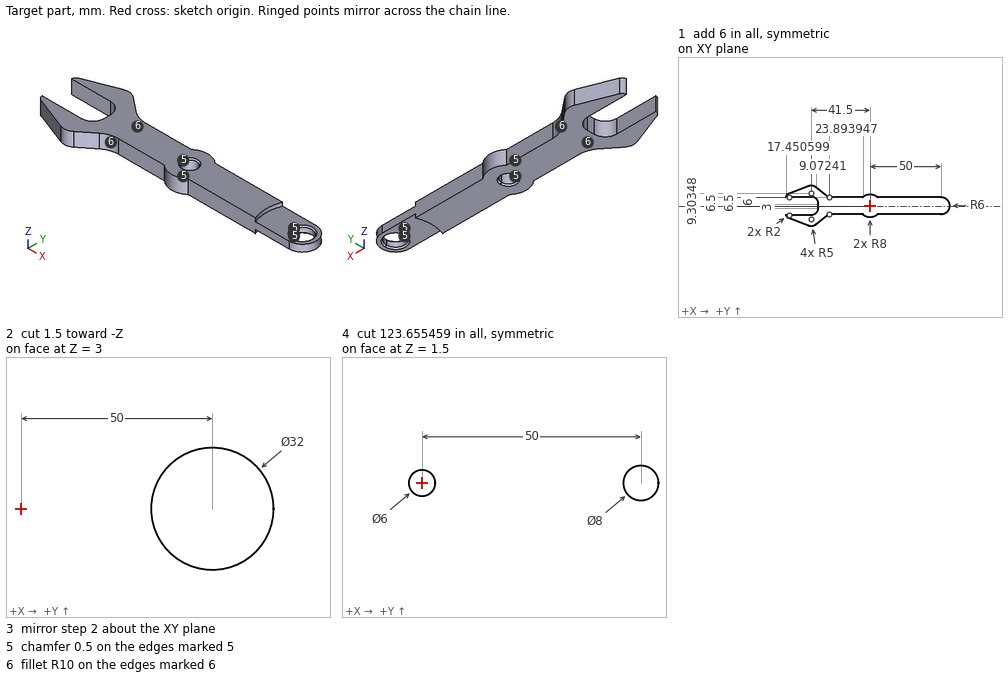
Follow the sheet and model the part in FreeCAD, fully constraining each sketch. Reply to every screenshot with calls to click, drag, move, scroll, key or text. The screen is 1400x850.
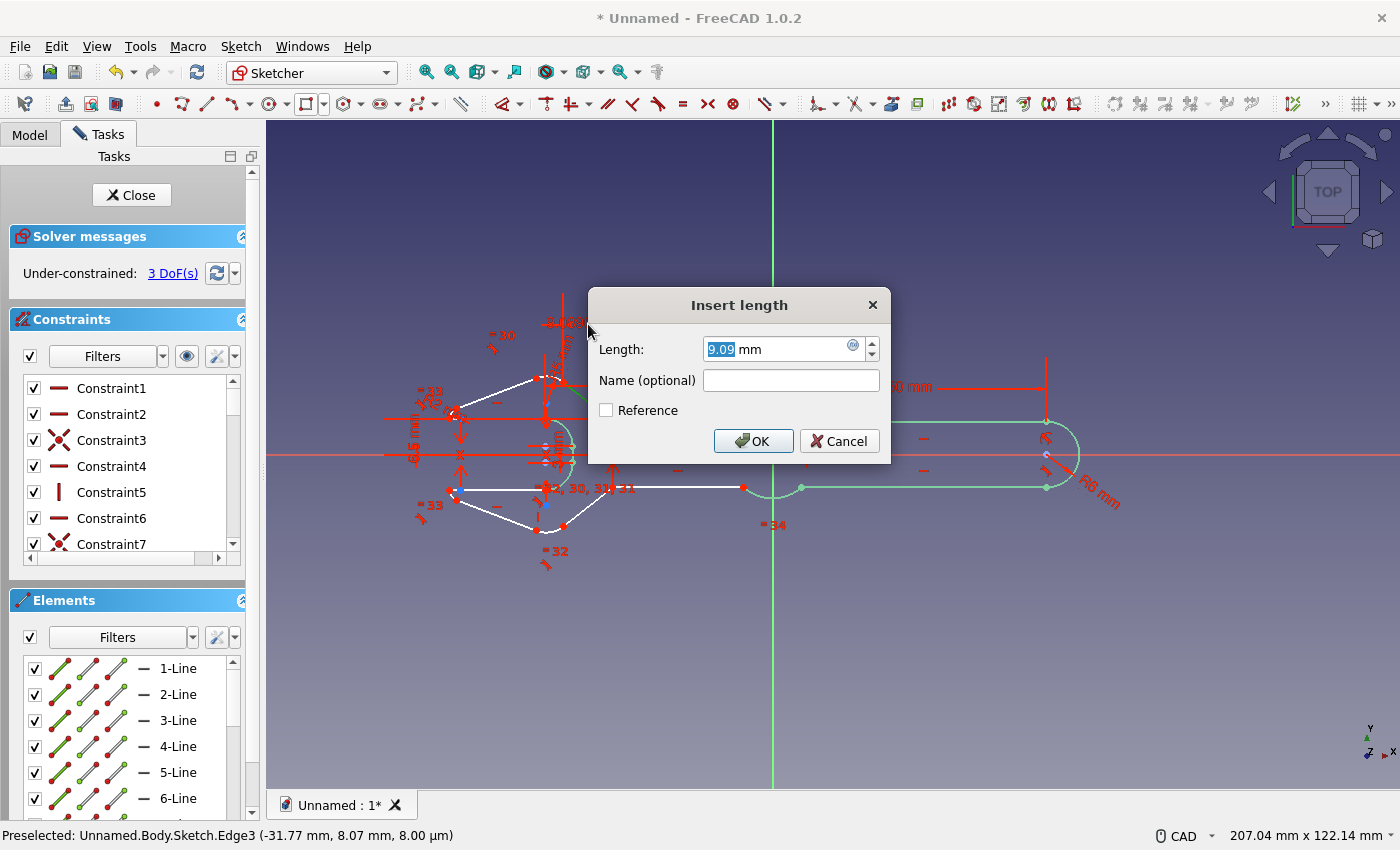
text(9.07241)
key(Return)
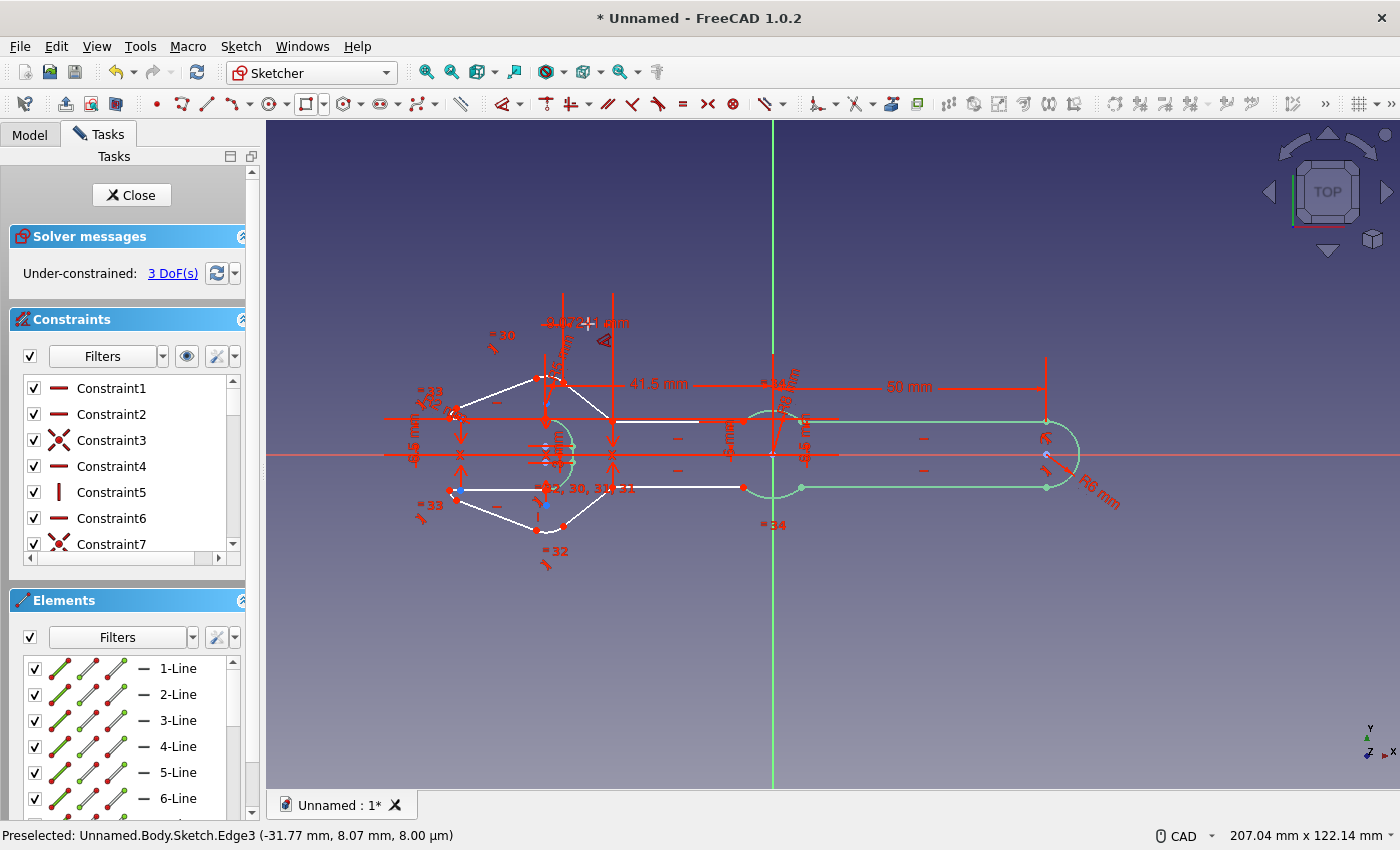
click(546, 404)
click(488, 441)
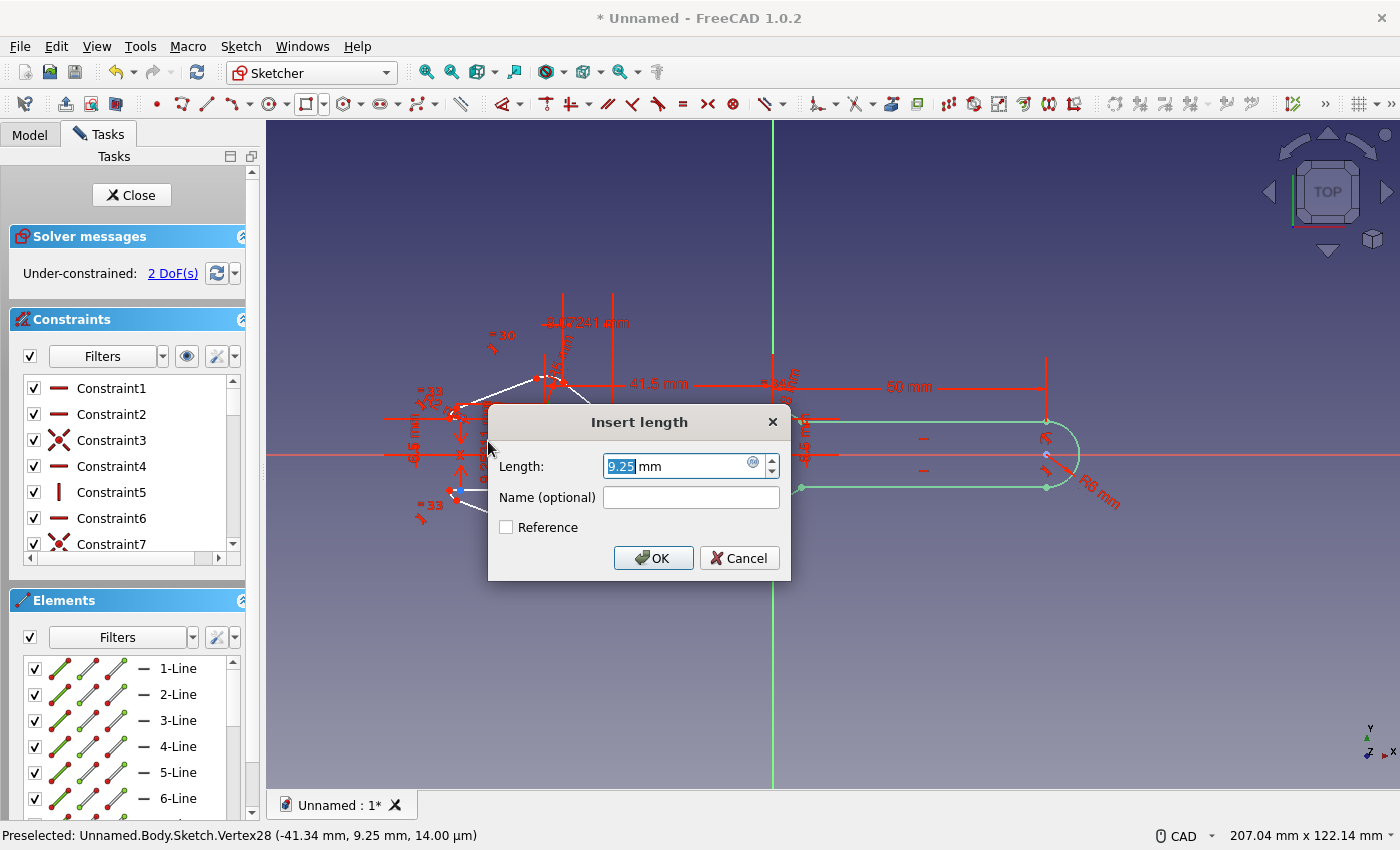
text(9.30348)
key(Return)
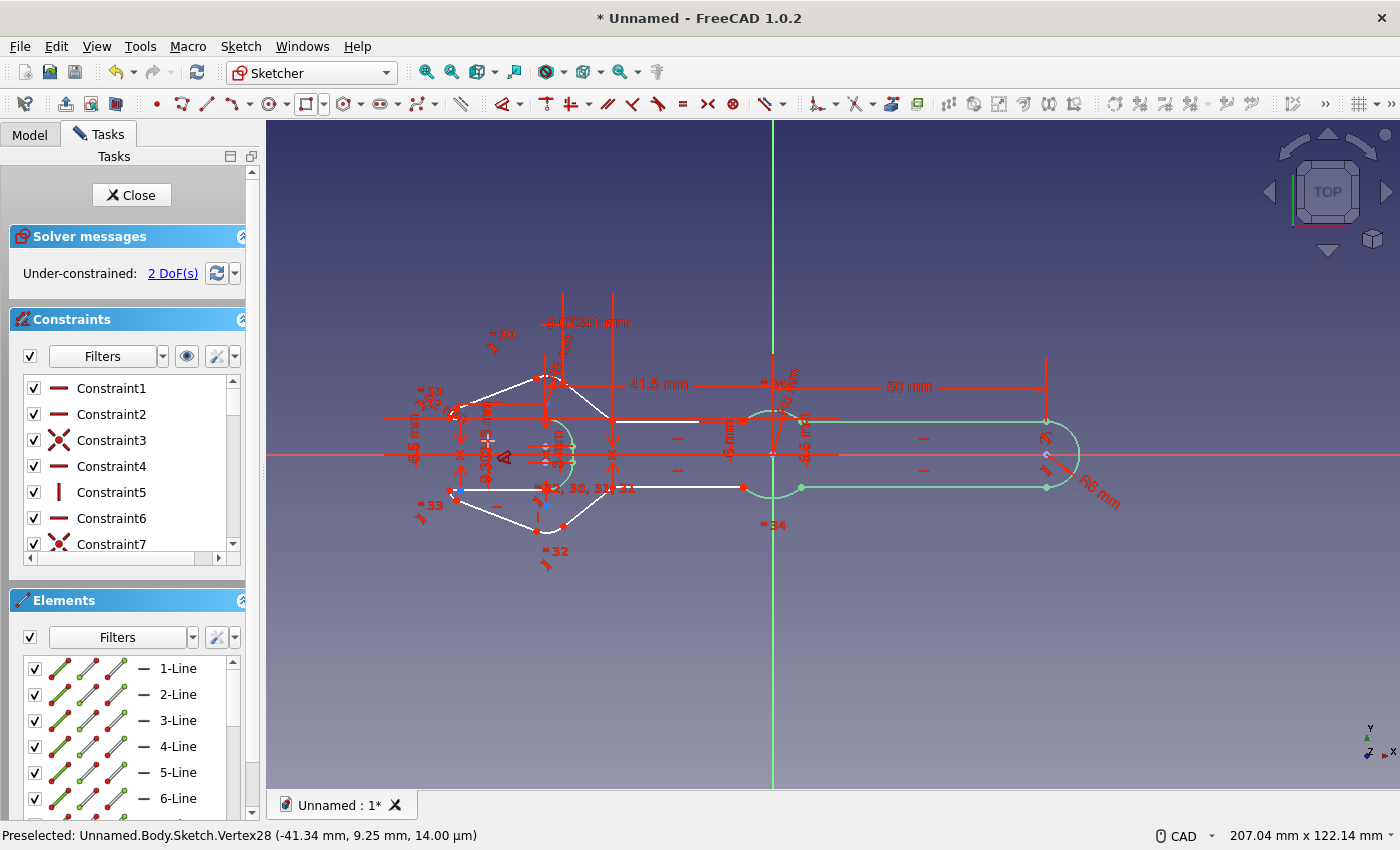
click(704, 422)
click(678, 364)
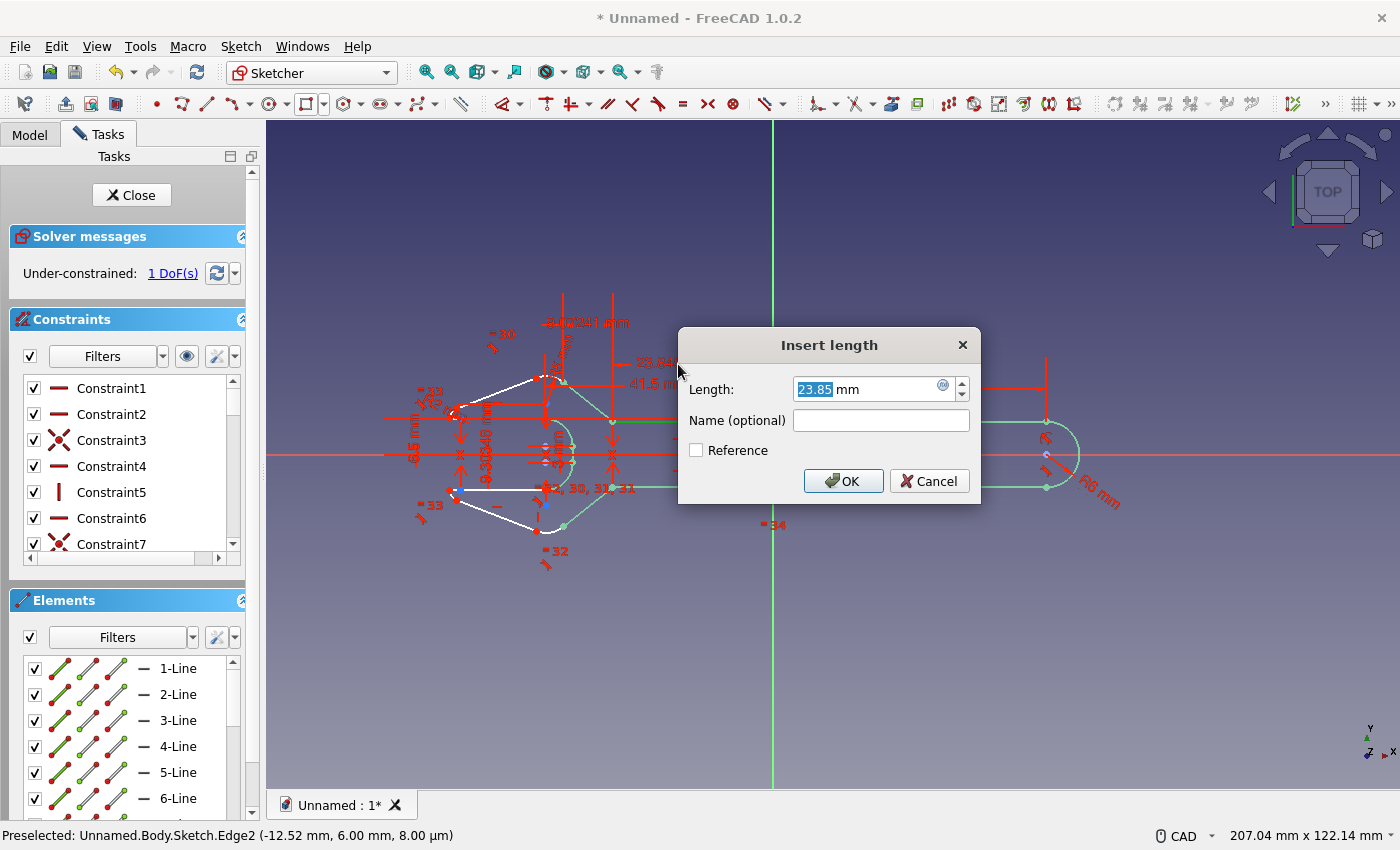
text(23.893947)
key(Return)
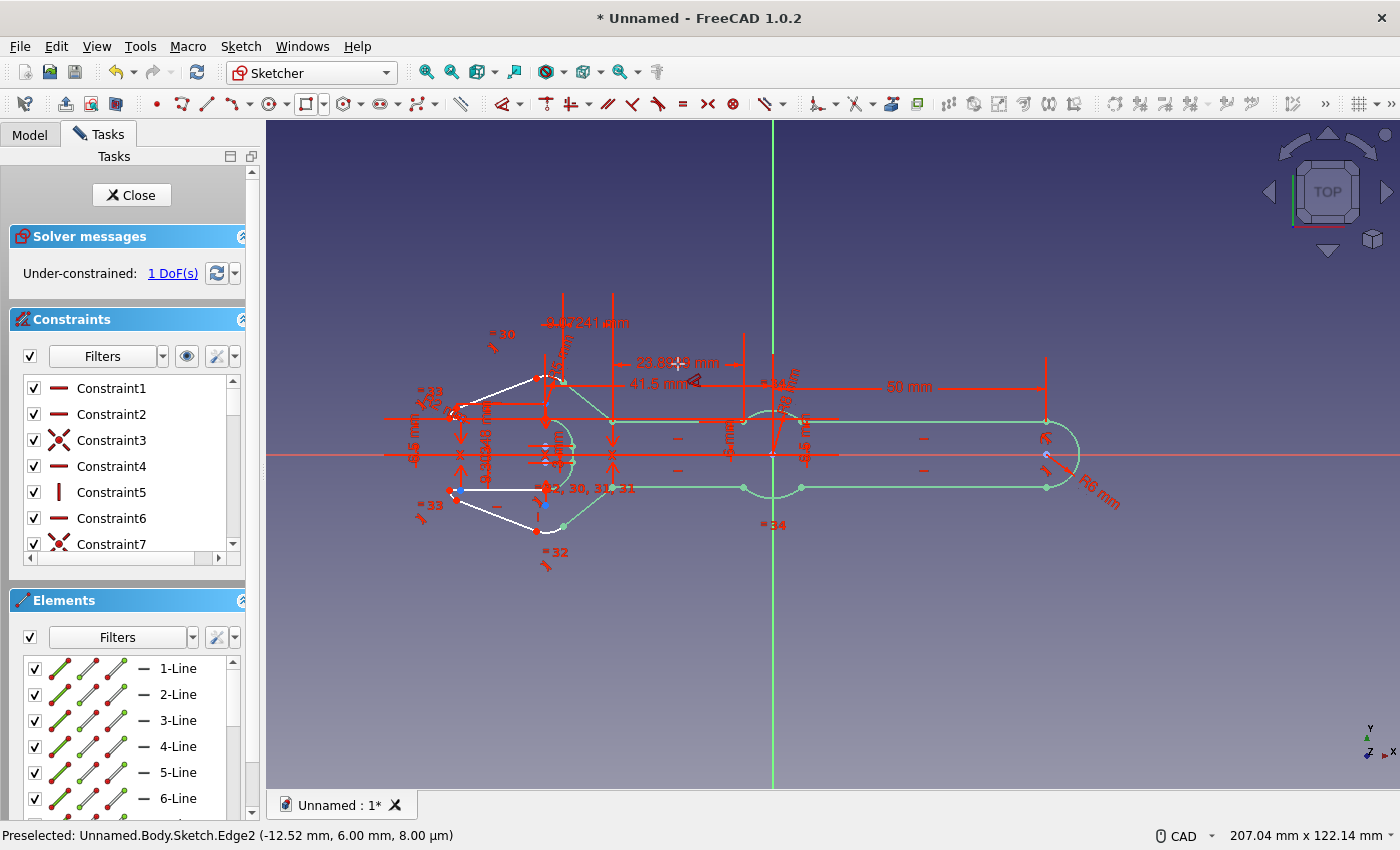
click(479, 419)
click(476, 385)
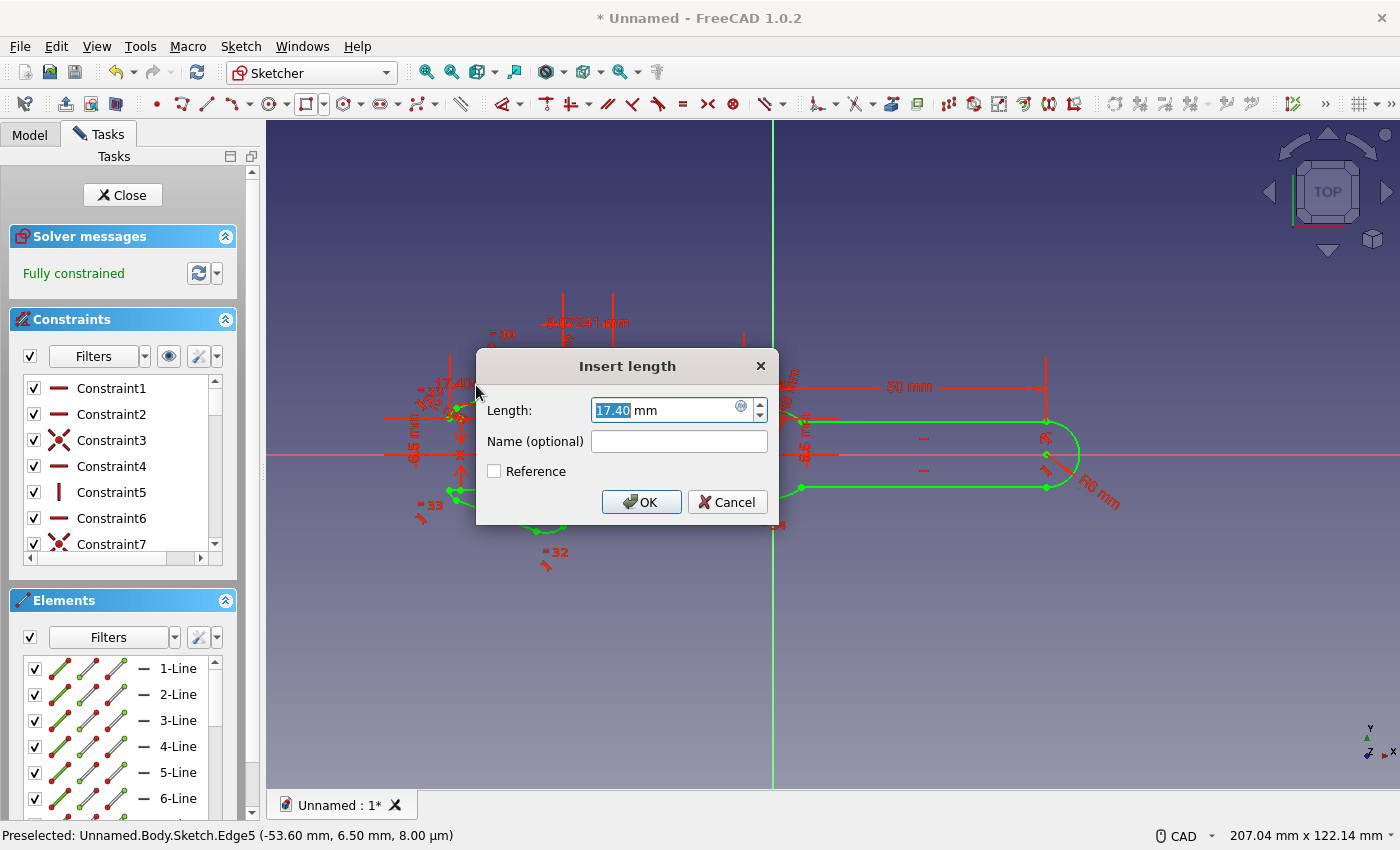
text(17.450599)
key(Return)
key(Escape)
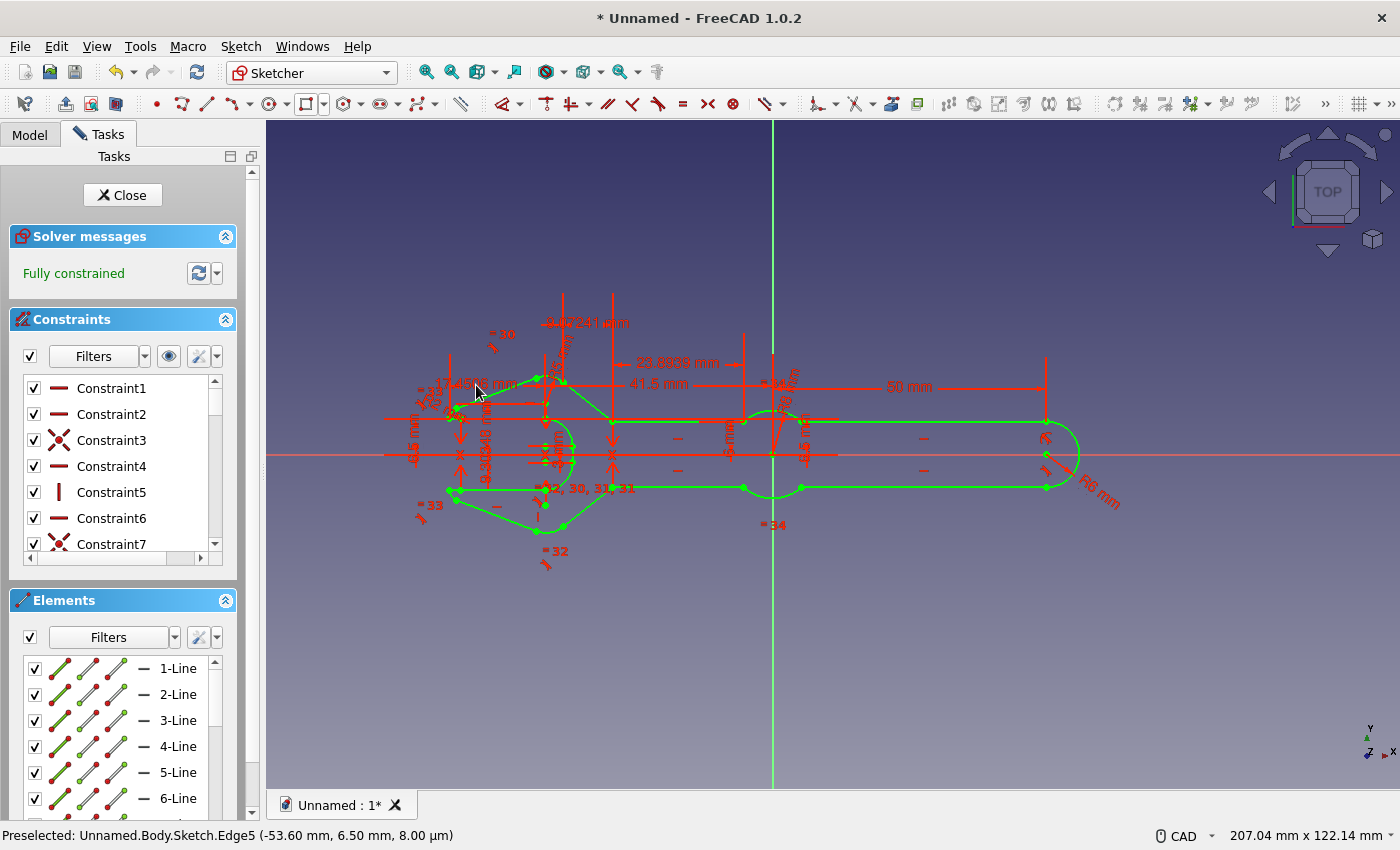
click(123, 195)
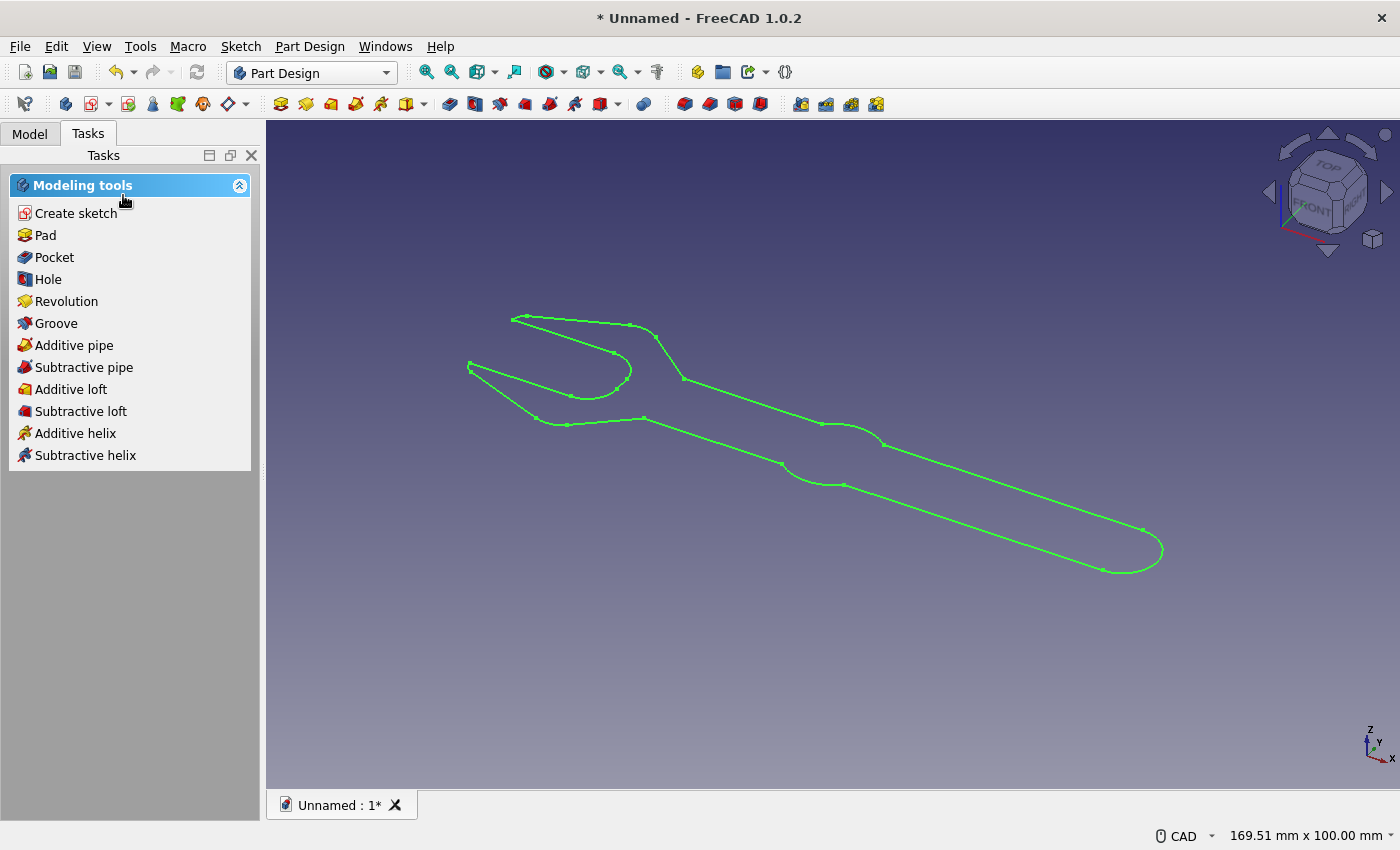
click(281, 104)